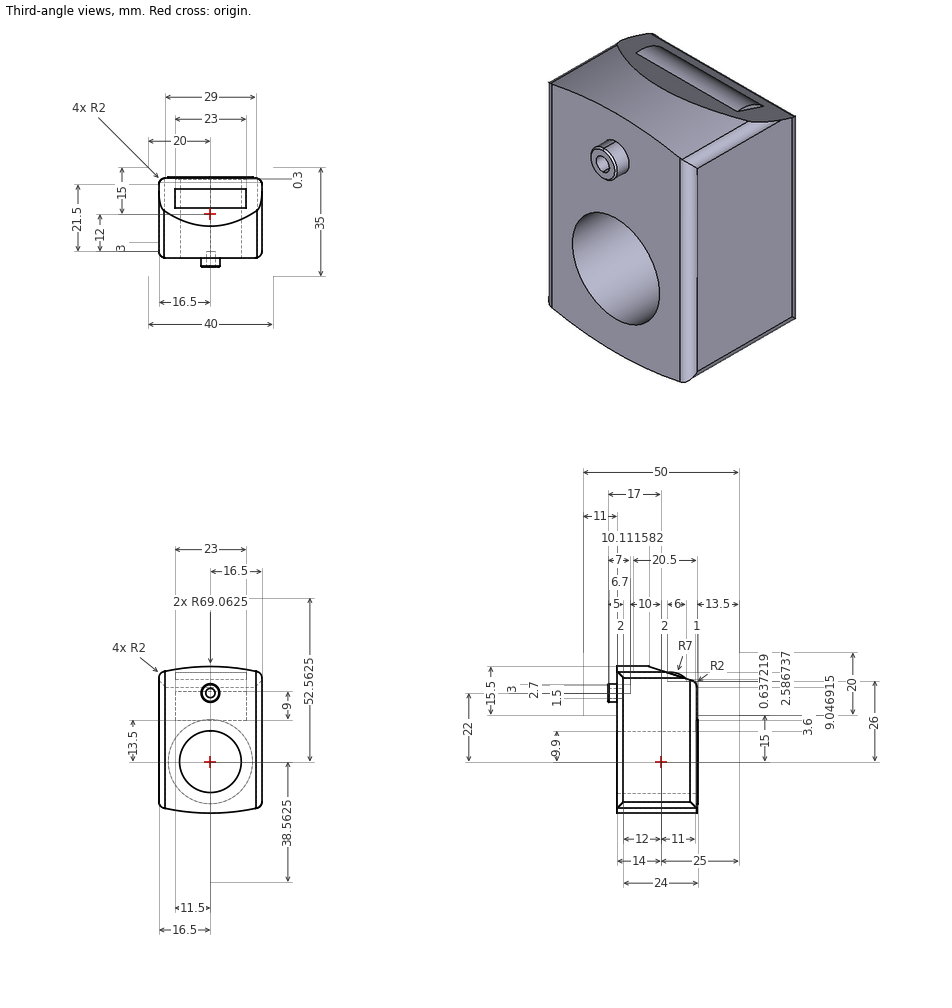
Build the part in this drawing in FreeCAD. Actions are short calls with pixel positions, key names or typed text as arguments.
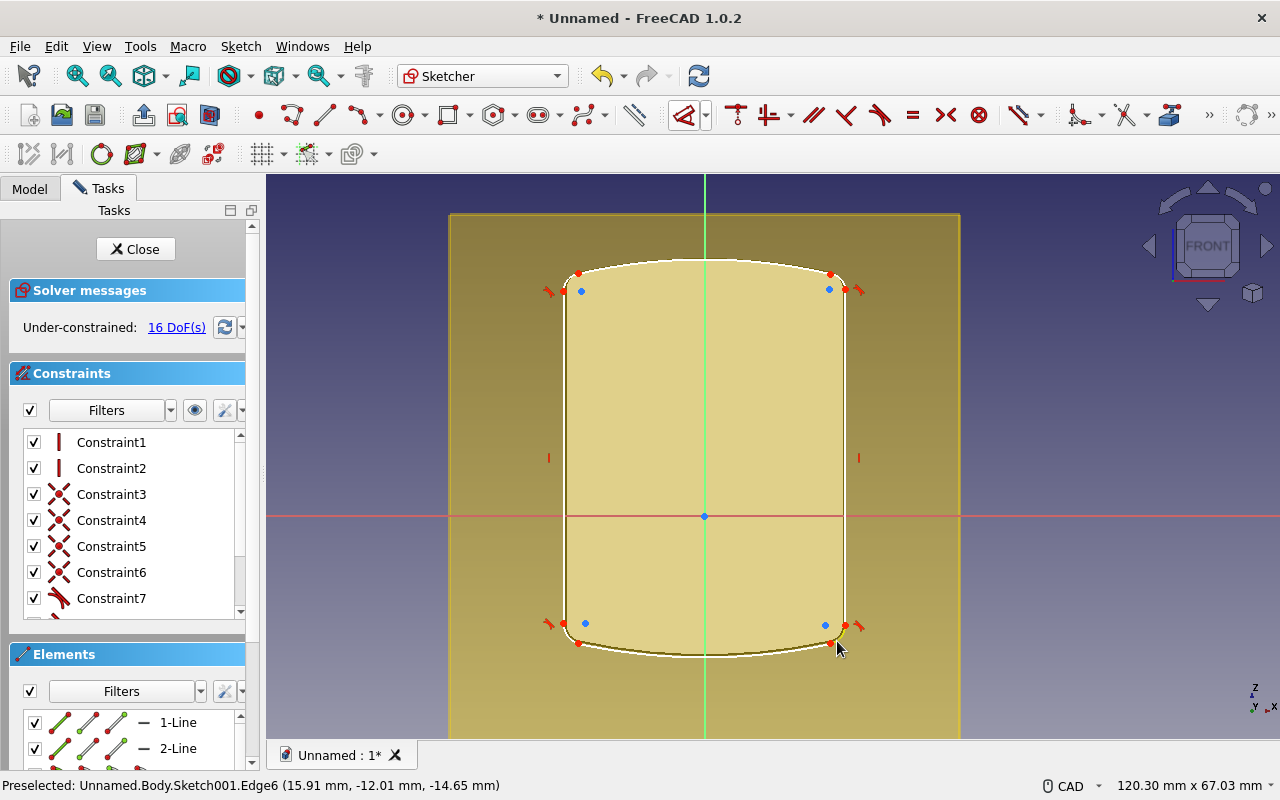
scroll(572, 277, up, 4)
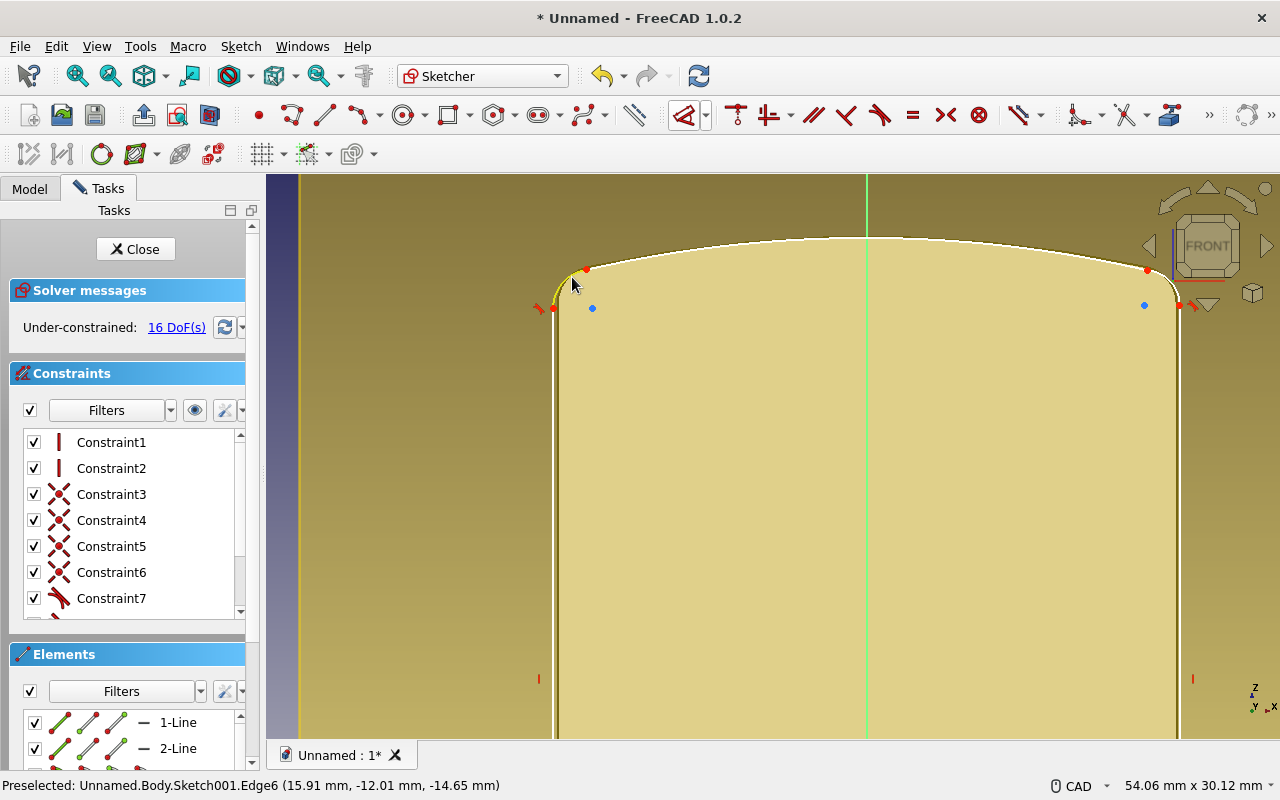
click(571, 276)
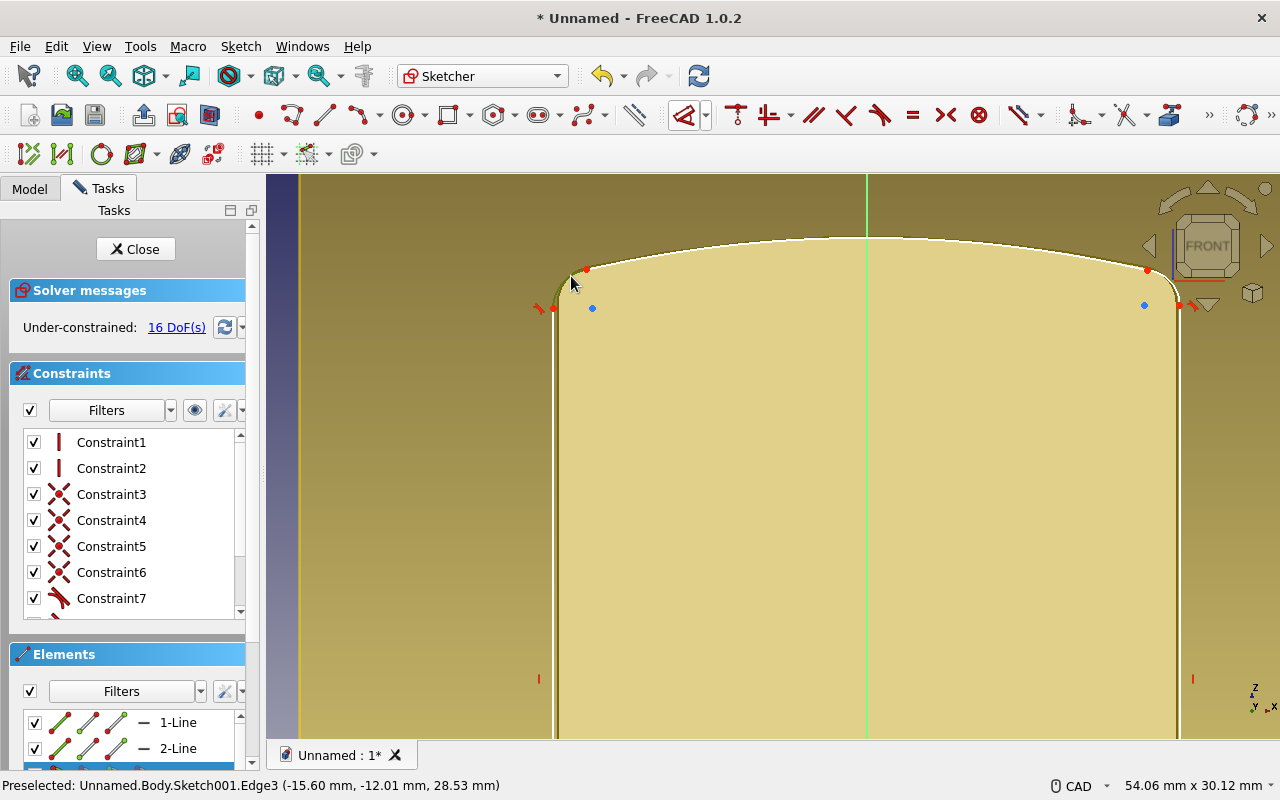
click(980, 243)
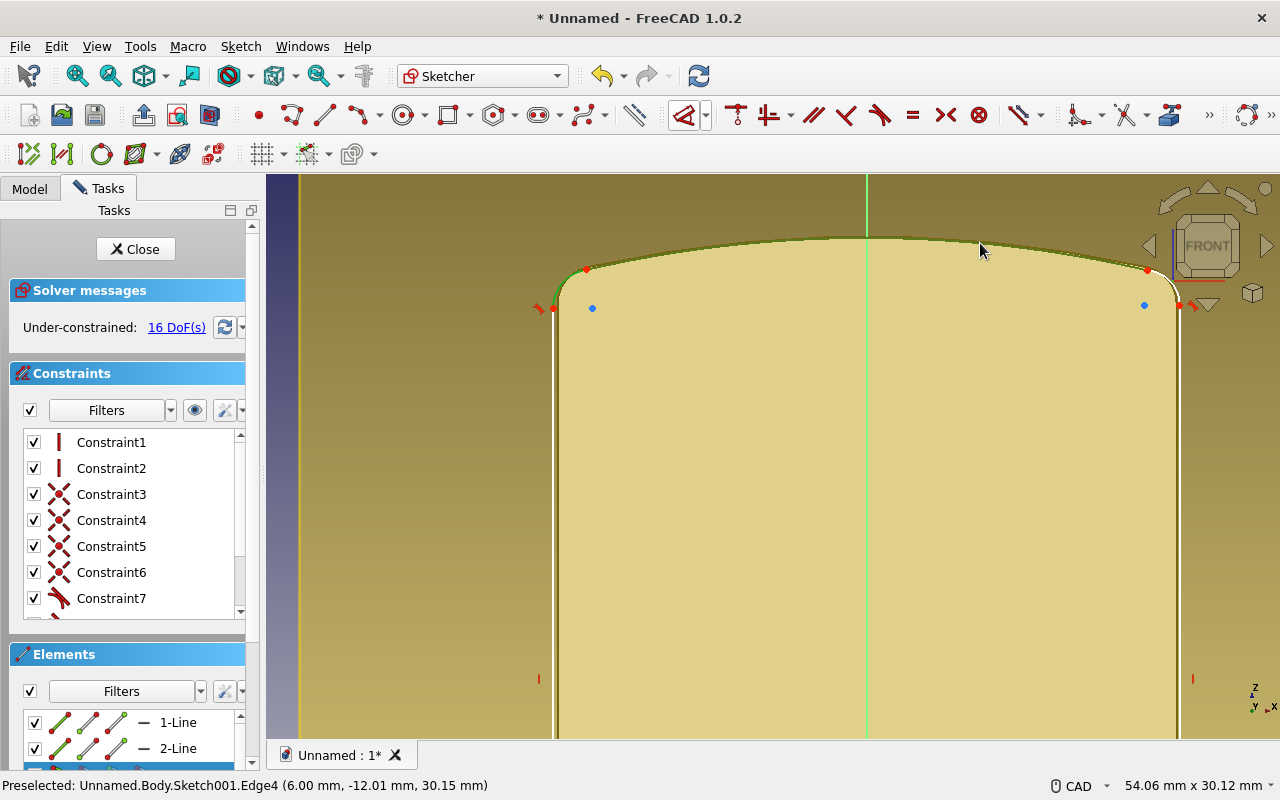
click(880, 116)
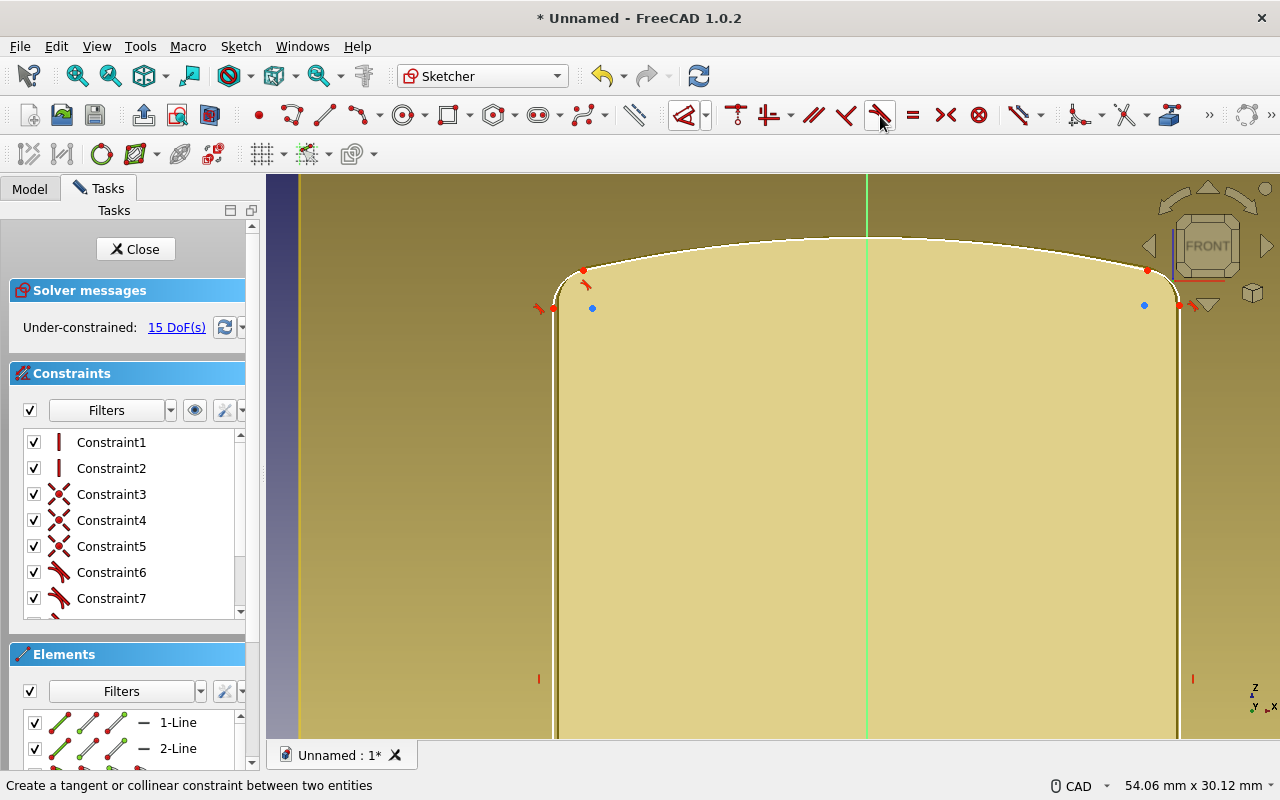
click(979, 243)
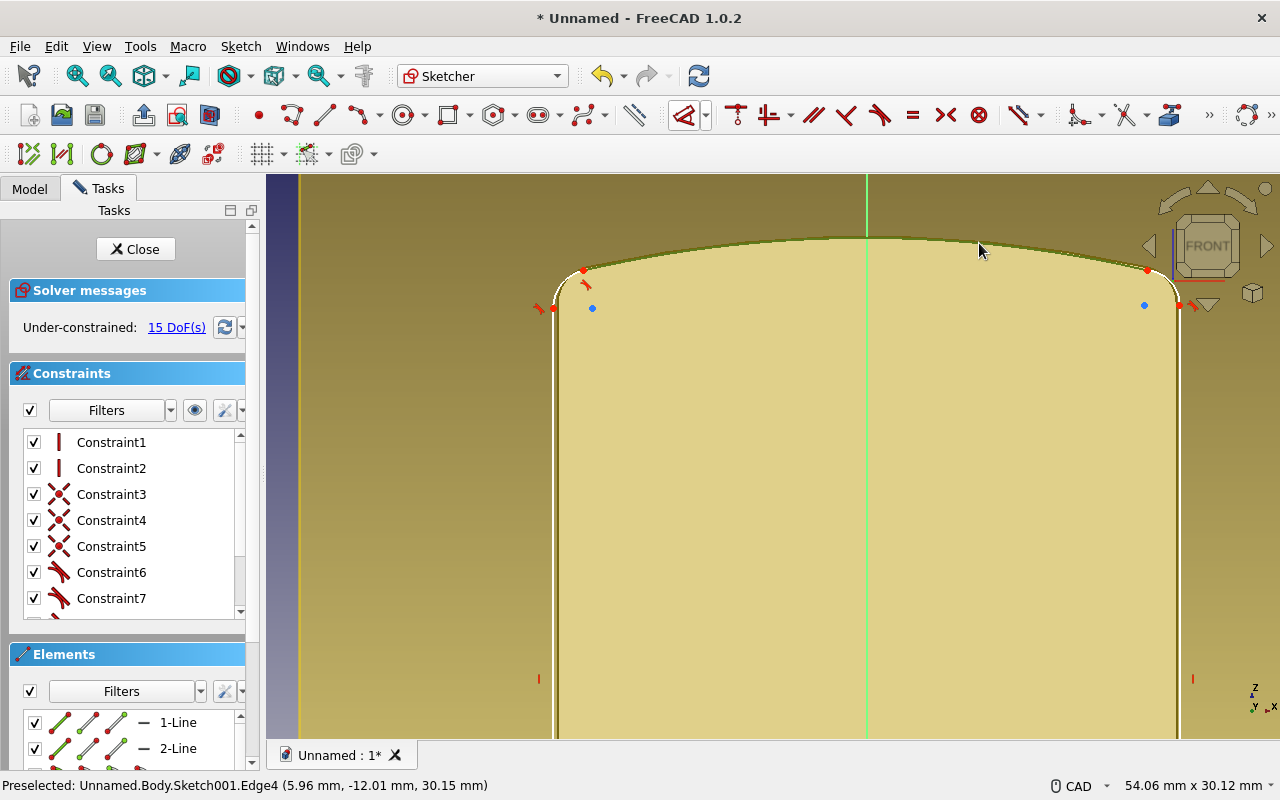
scroll(572, 276, down, 4)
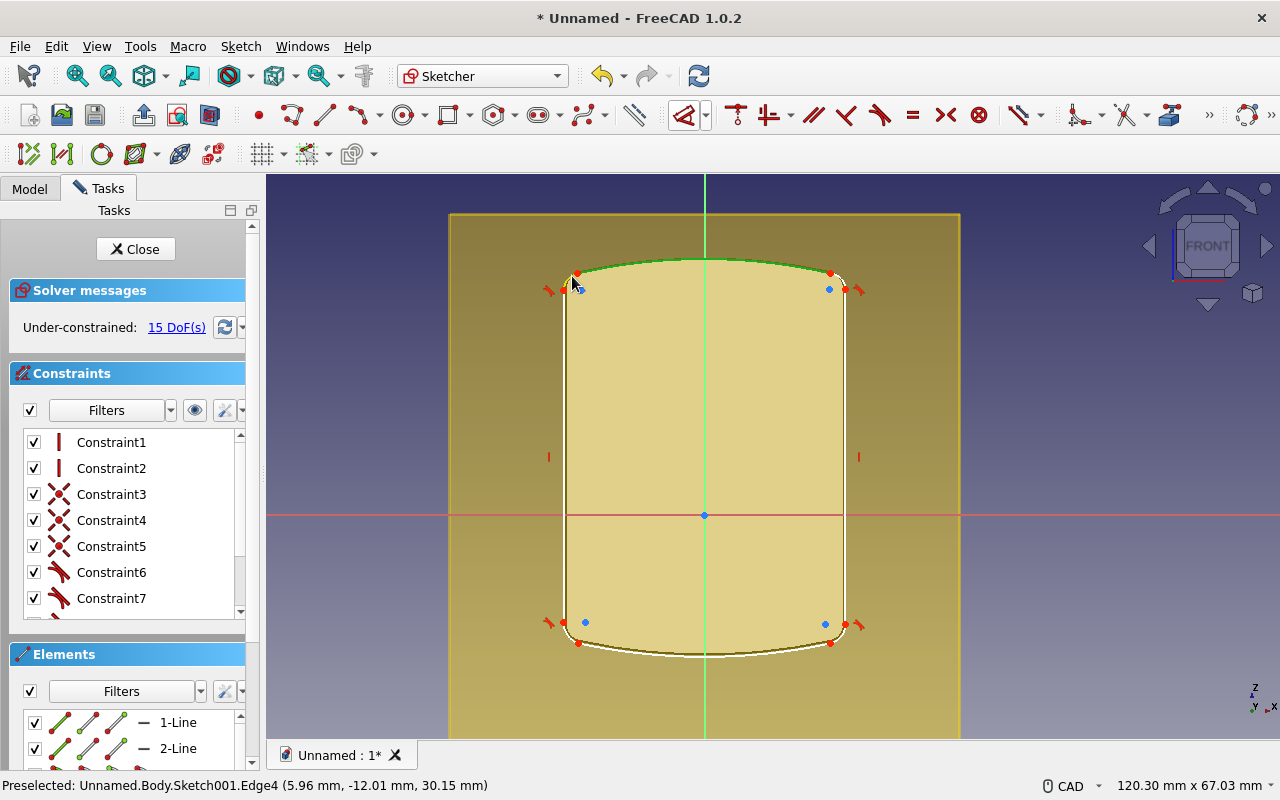
scroll(844, 282, up, 4)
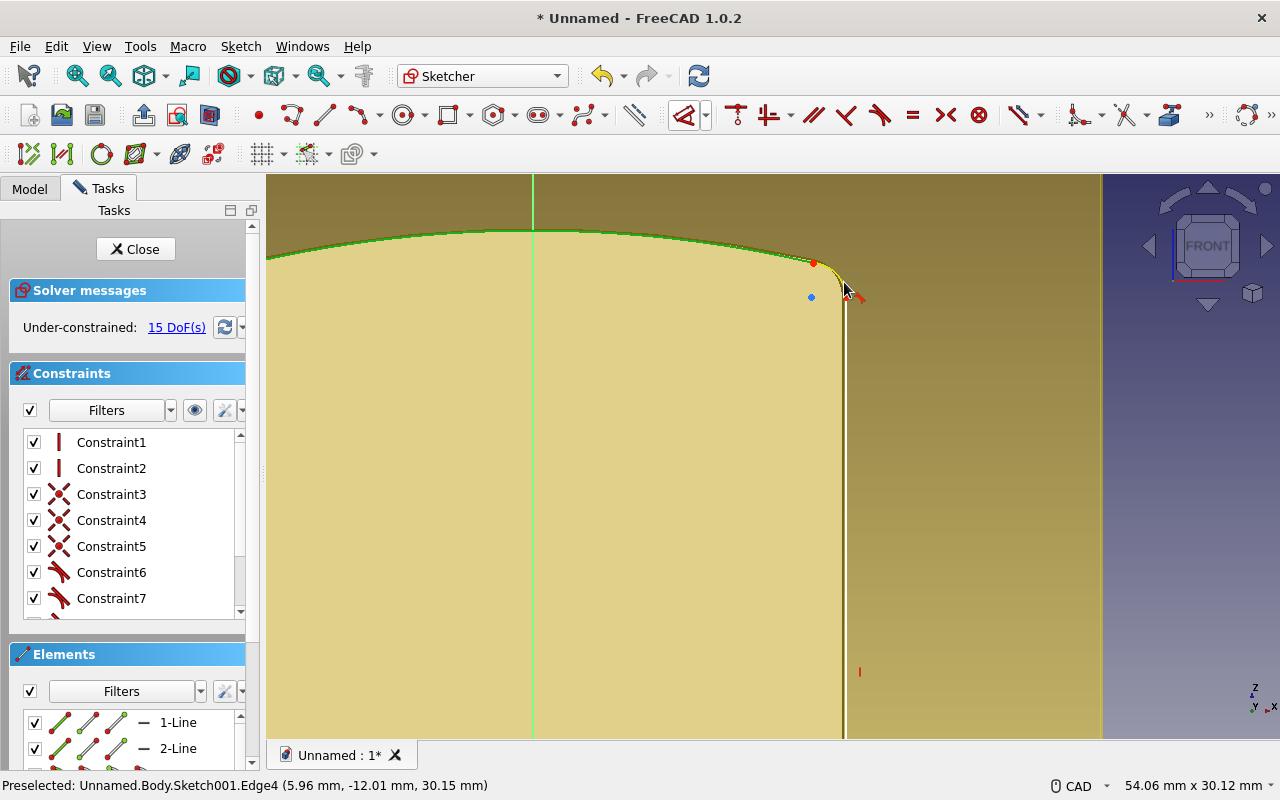
click(843, 283)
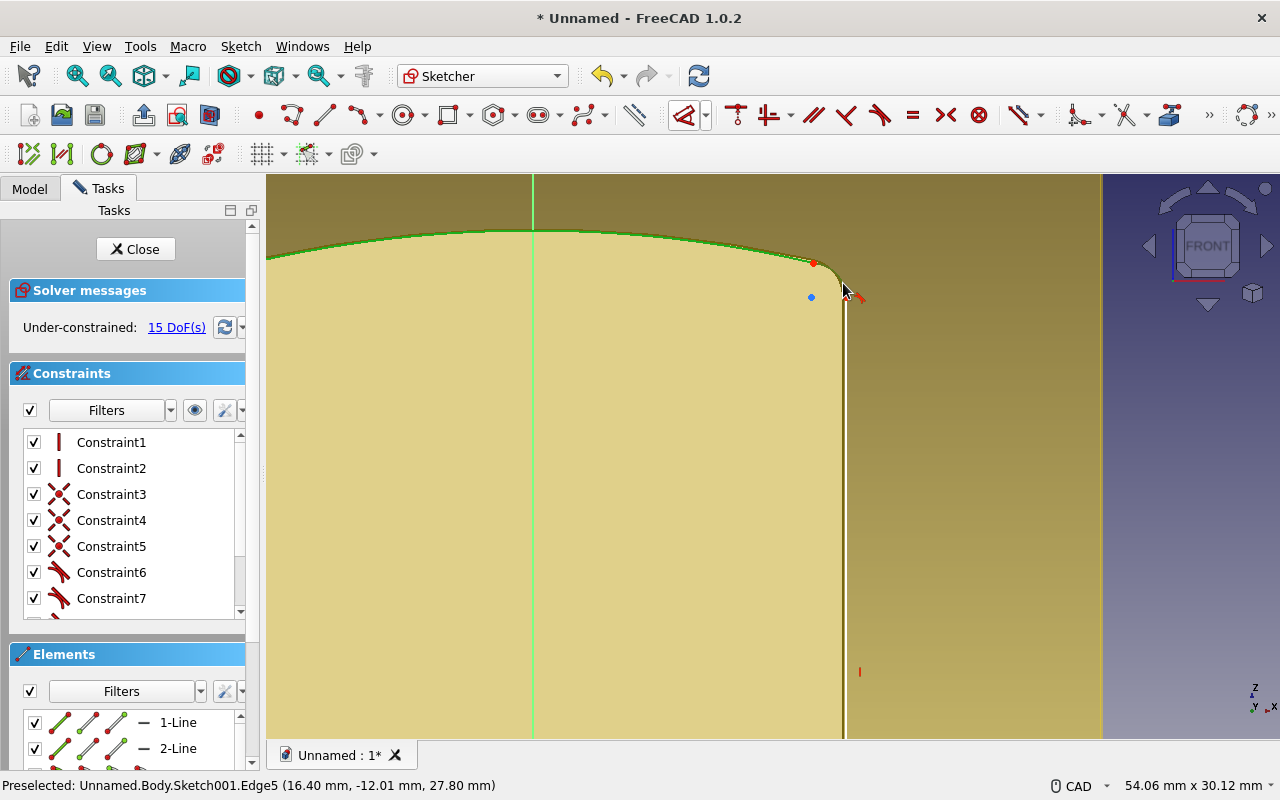
click(880, 116)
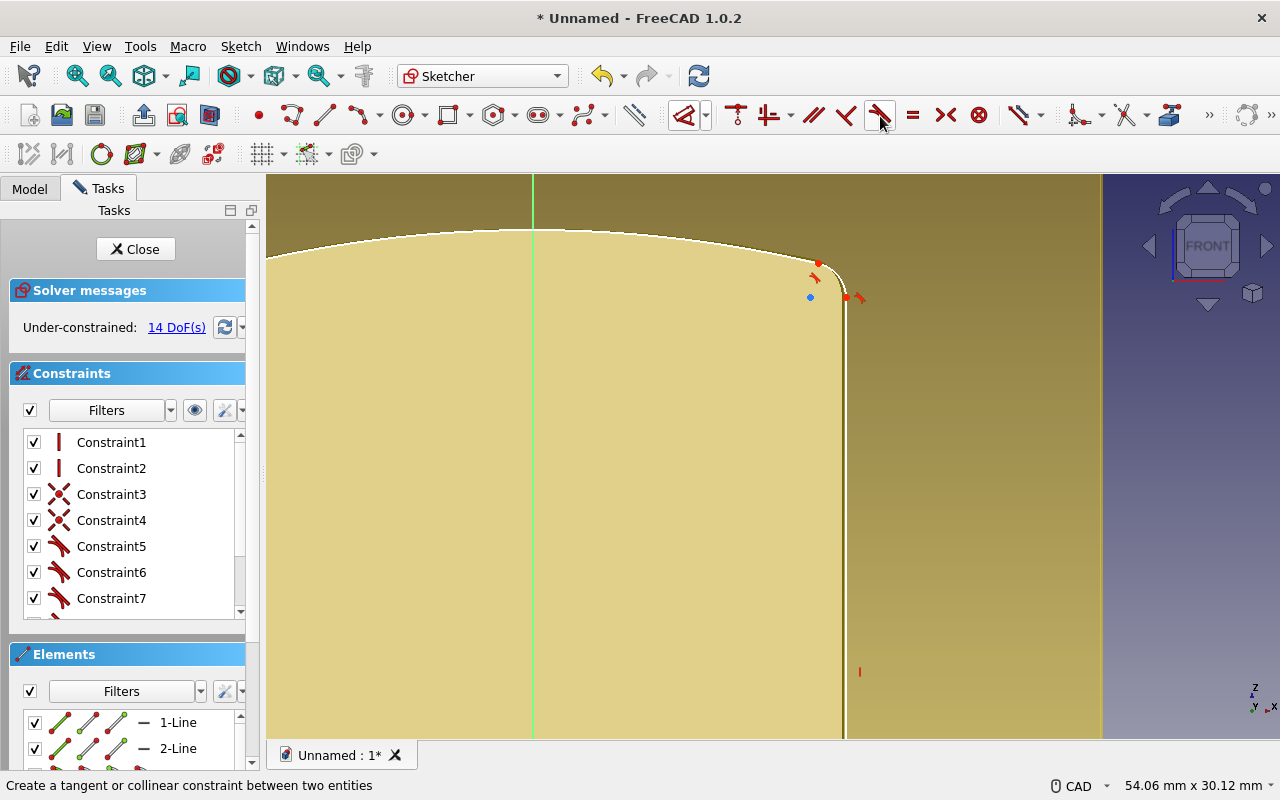
scroll(844, 282, down, 4)